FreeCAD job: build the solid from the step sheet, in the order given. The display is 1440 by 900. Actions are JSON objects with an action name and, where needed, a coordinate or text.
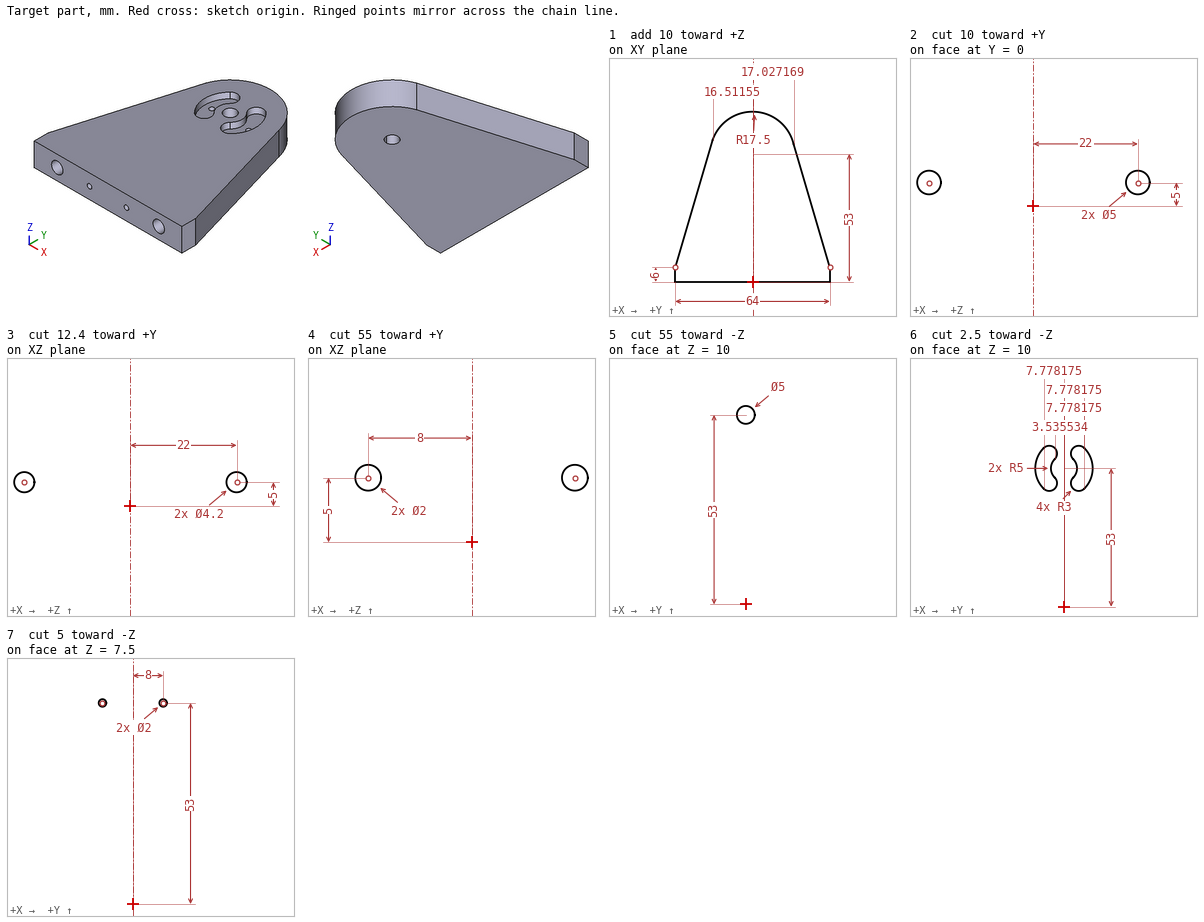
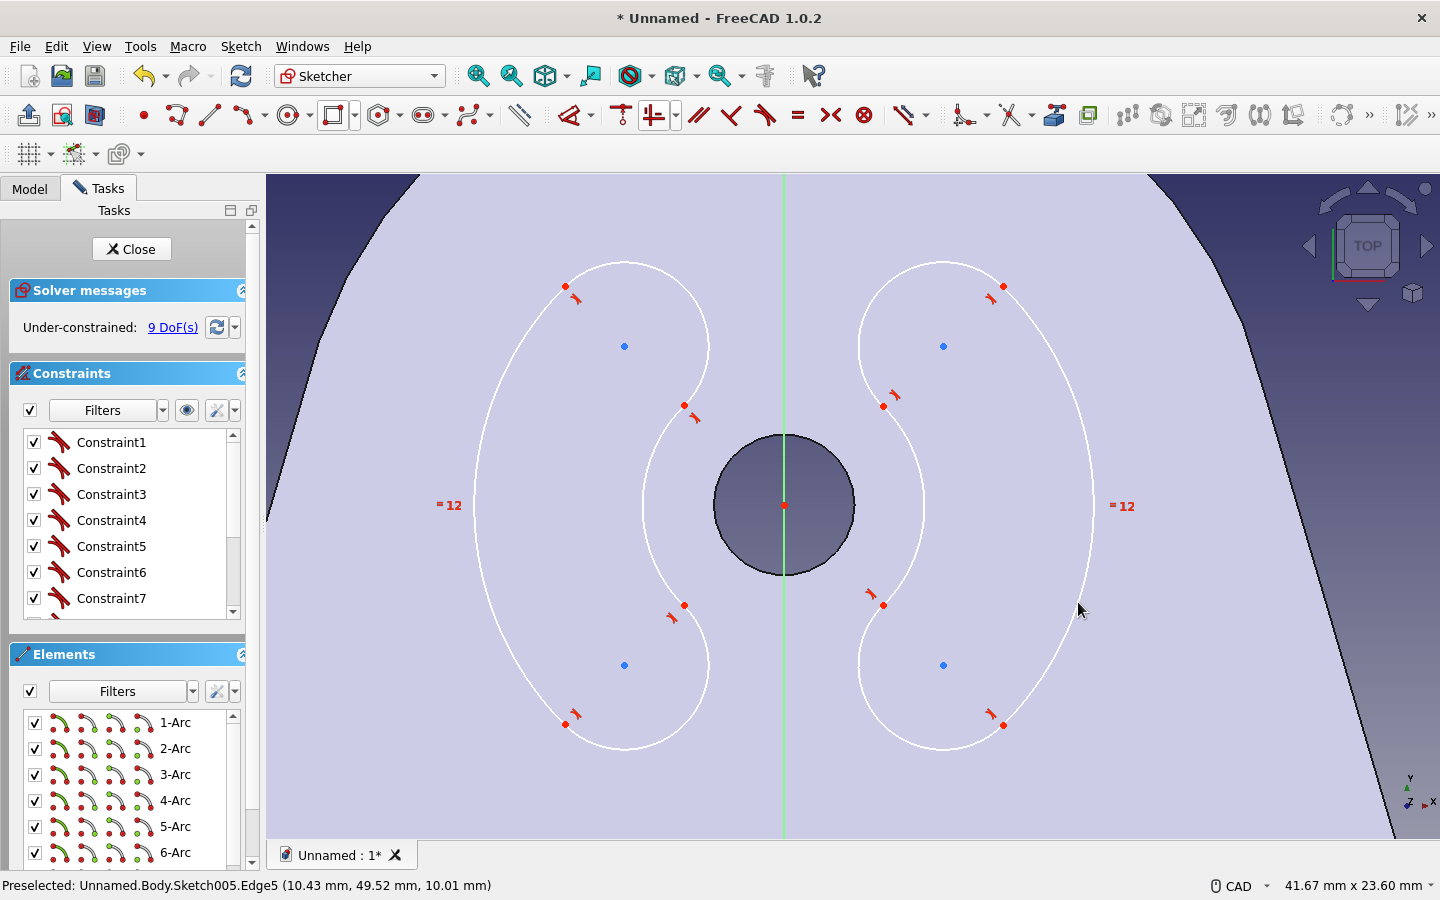
{"action": "left_click", "coordinate": [638, 749]}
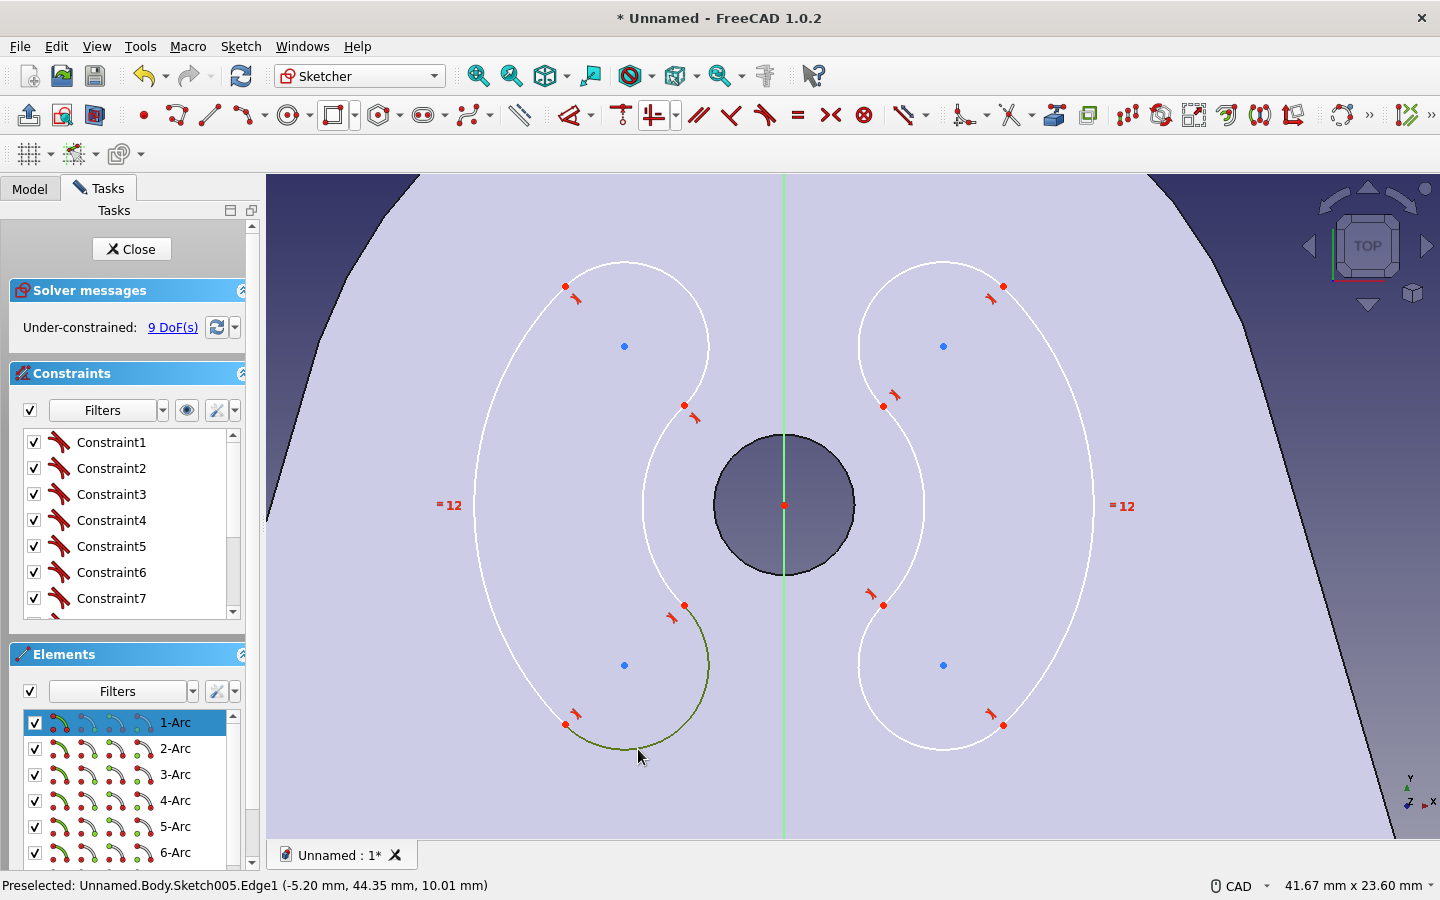
{"action": "left_click", "coordinate": [930, 263]}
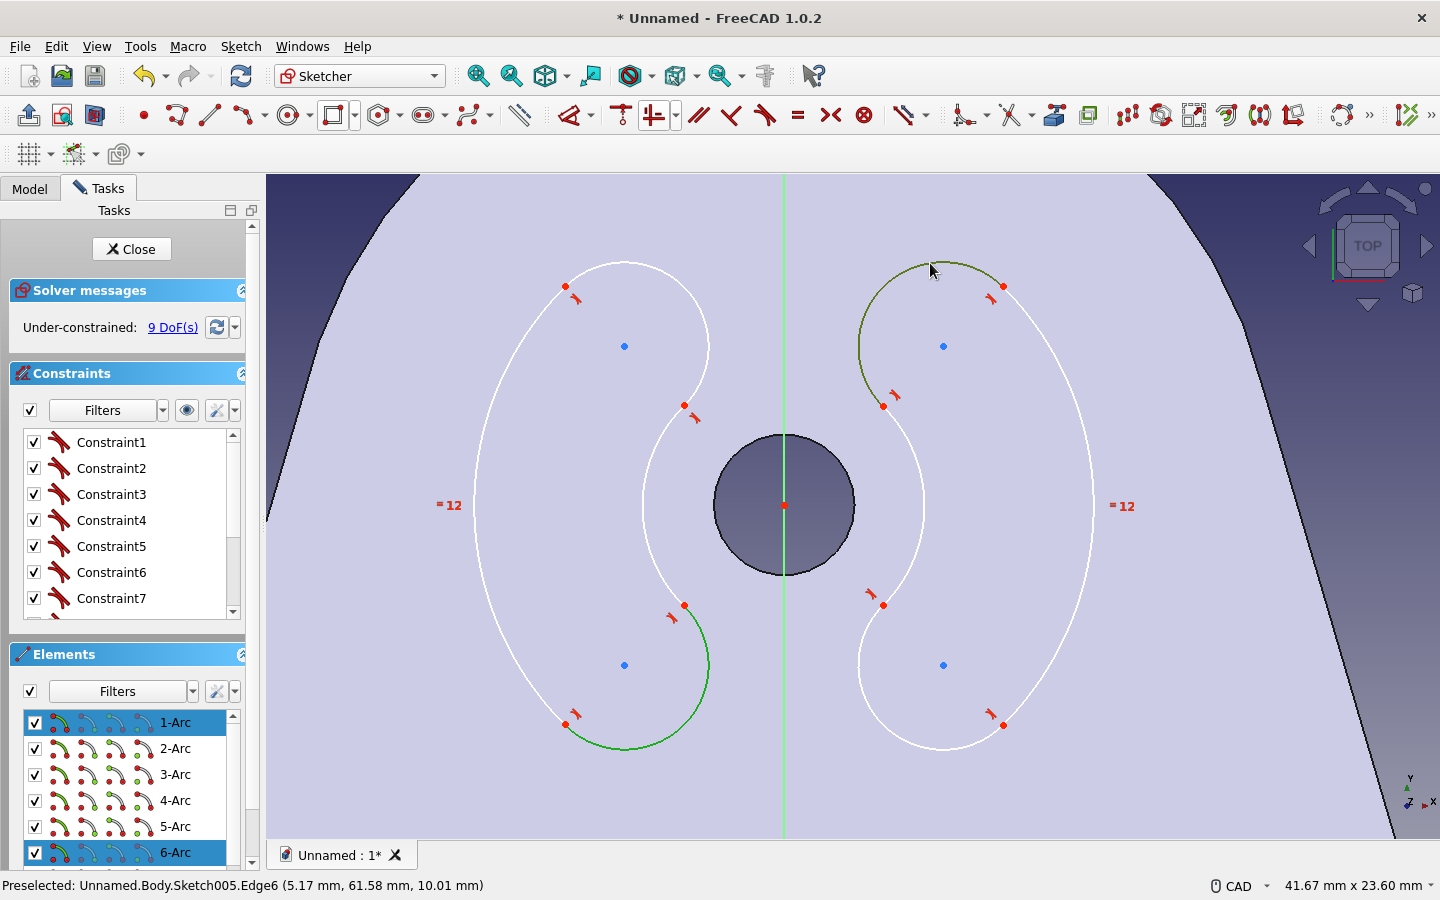
{"action": "key", "text": "e"}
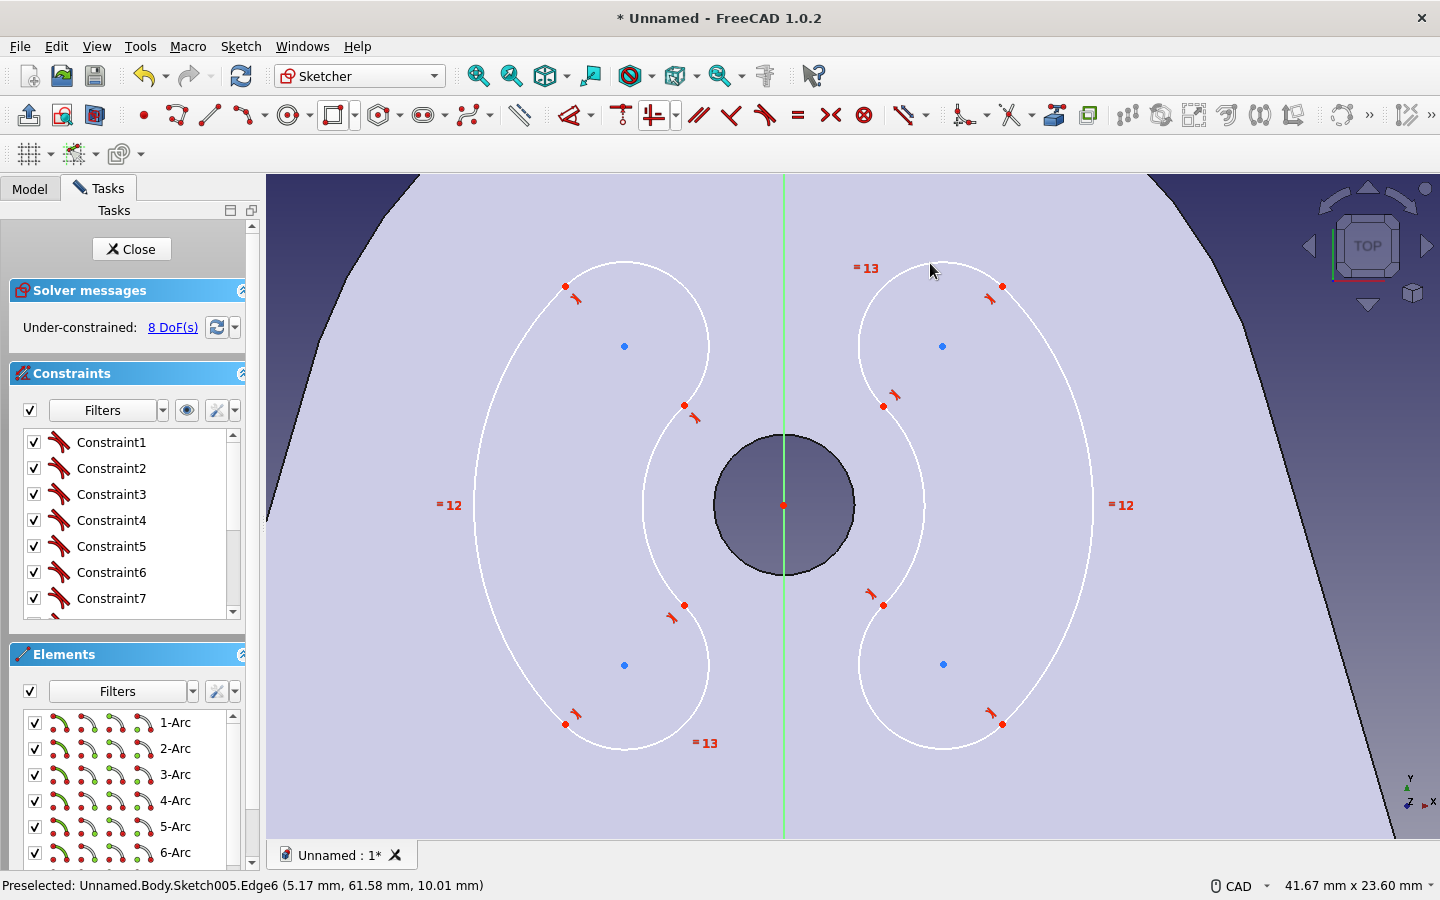
{"action": "left_click", "coordinate": [784, 506]}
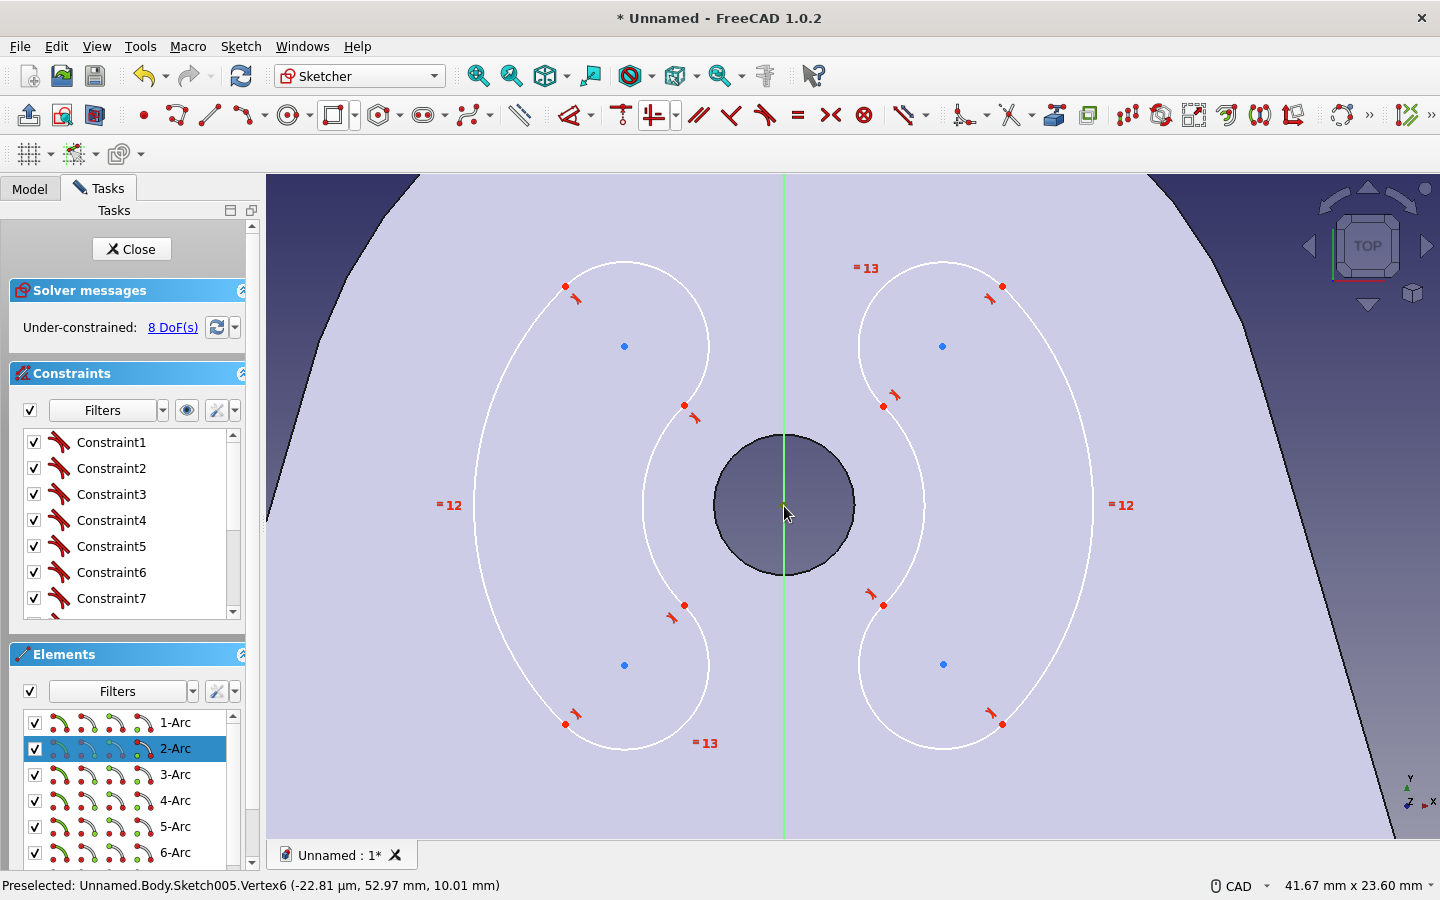
{"action": "left_click", "coordinate": [784, 768]}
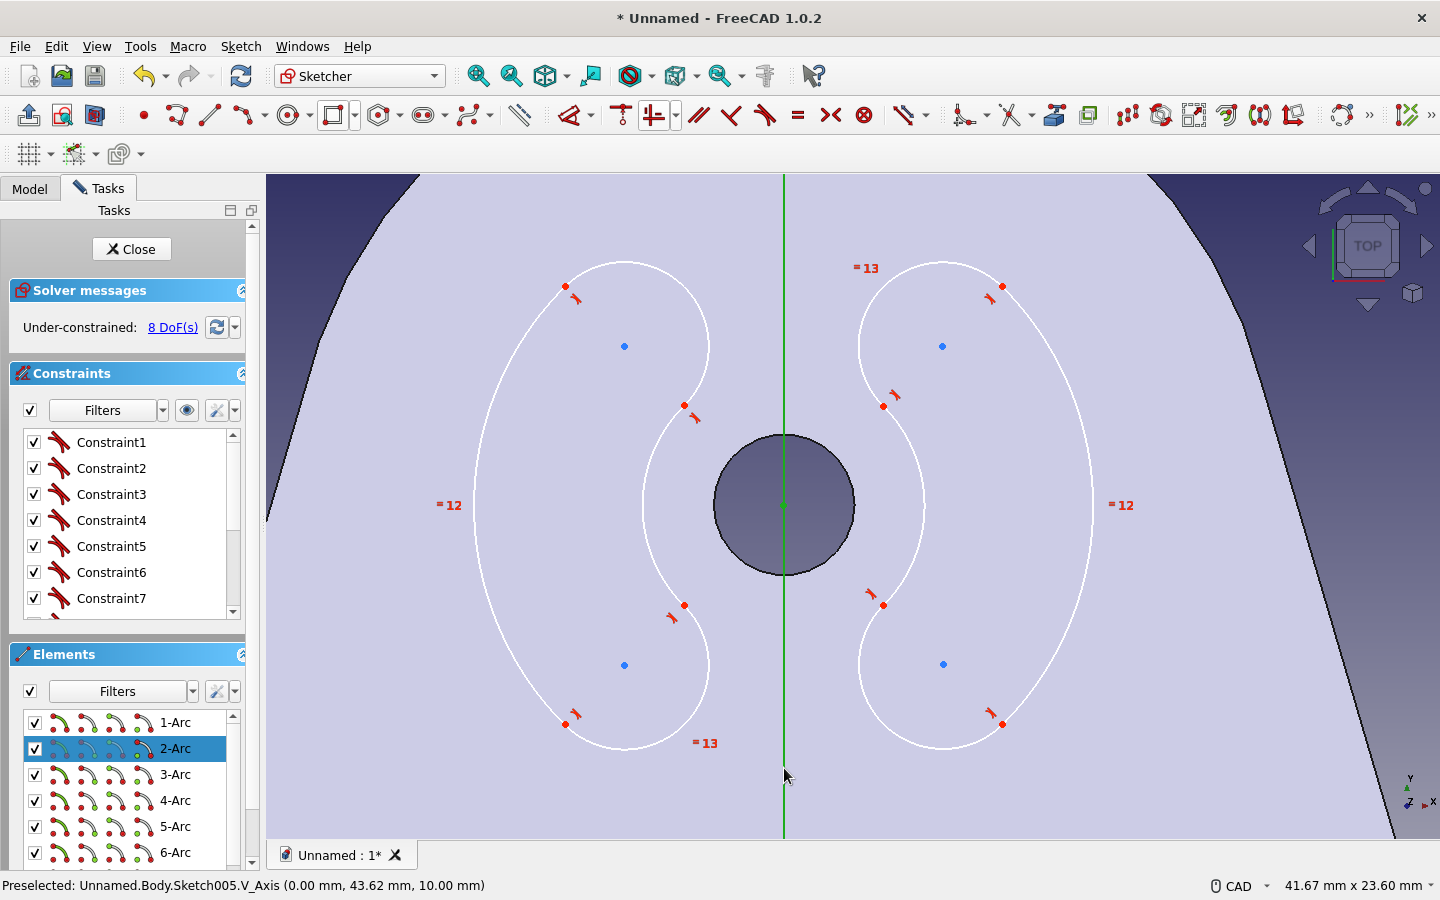
{"action": "left_click", "coordinate": [621, 116]}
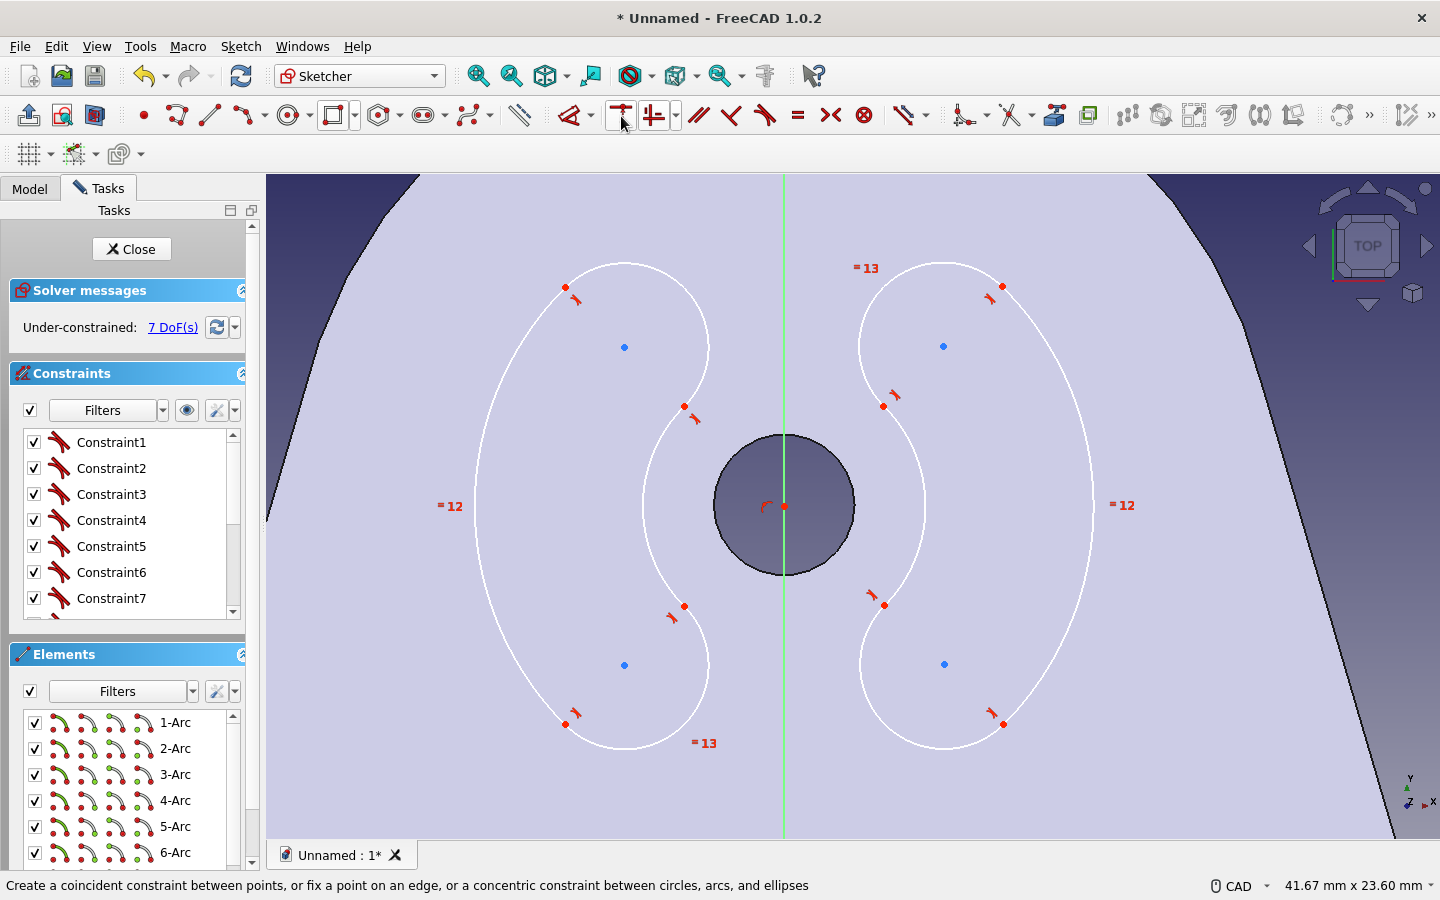
{"action": "left_click", "coordinate": [568, 116]}